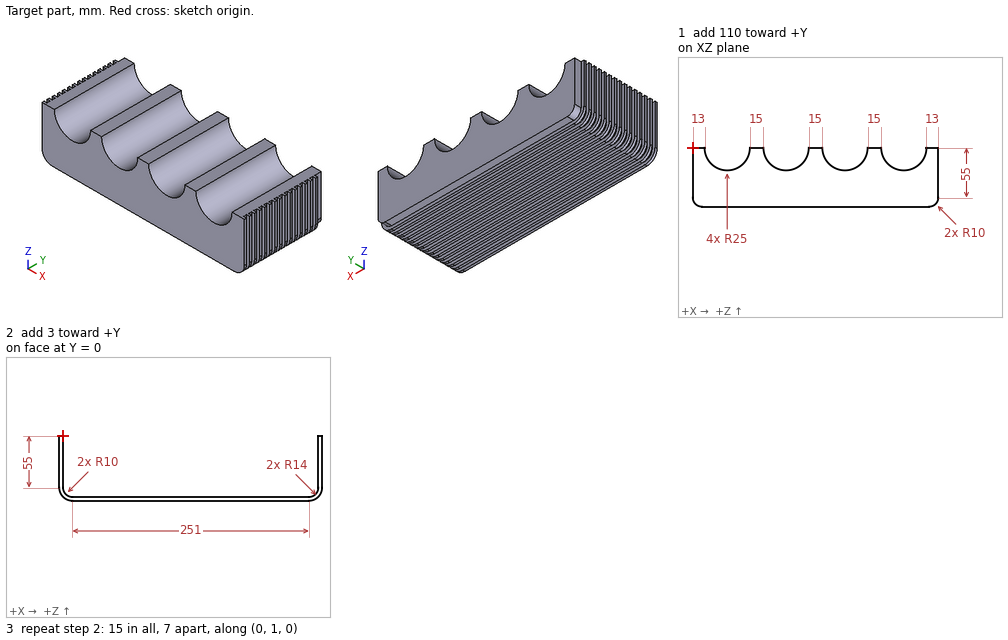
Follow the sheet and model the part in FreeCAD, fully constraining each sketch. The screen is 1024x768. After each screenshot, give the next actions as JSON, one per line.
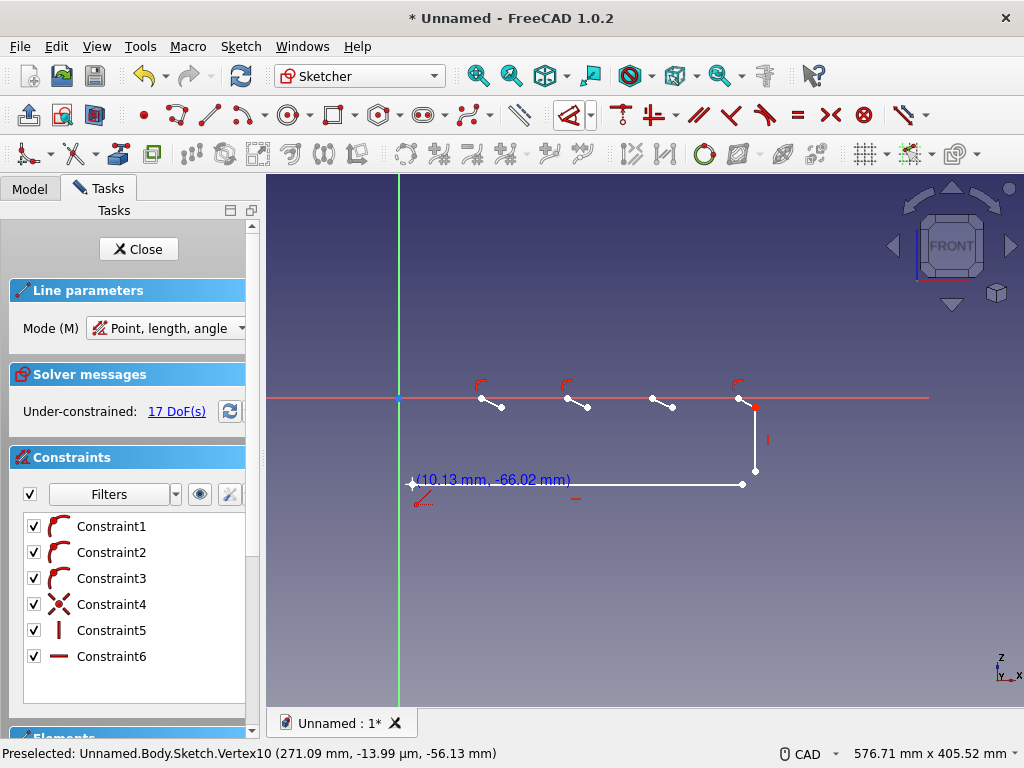
{"action": "key", "text": "g m"}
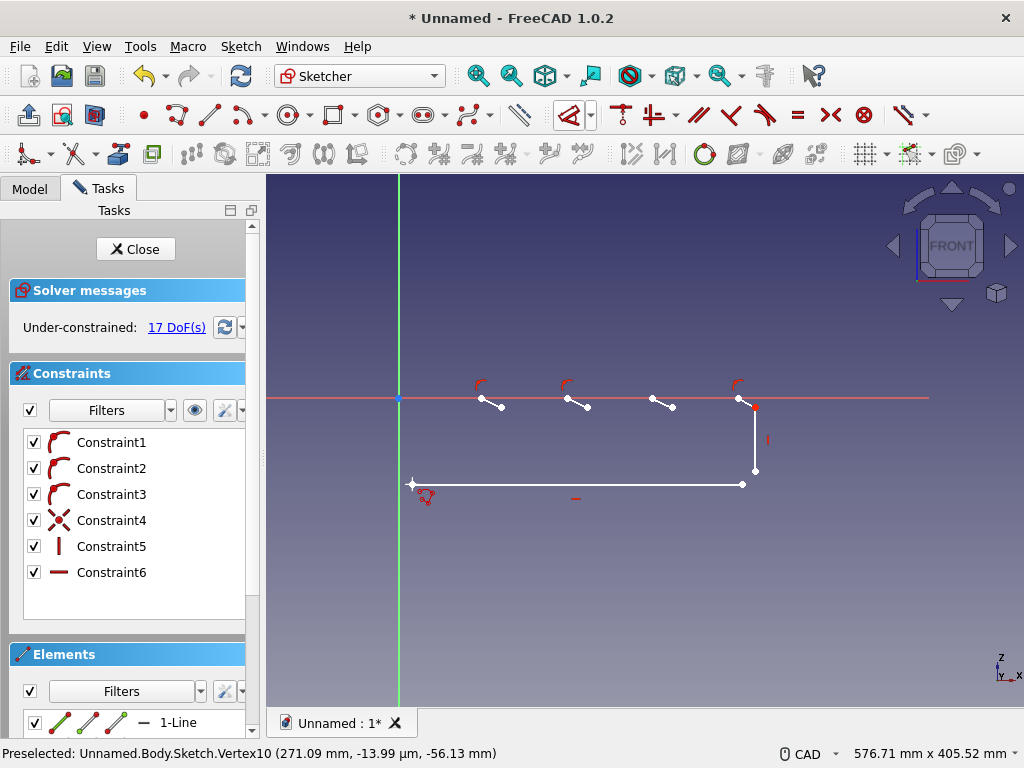
{"action": "left_click", "coordinate": [399, 471]}
{"action": "left_click", "coordinate": [399, 398]}
{"action": "left_click", "coordinate": [416, 407]}
{"action": "right_click", "coordinate": [416, 407]}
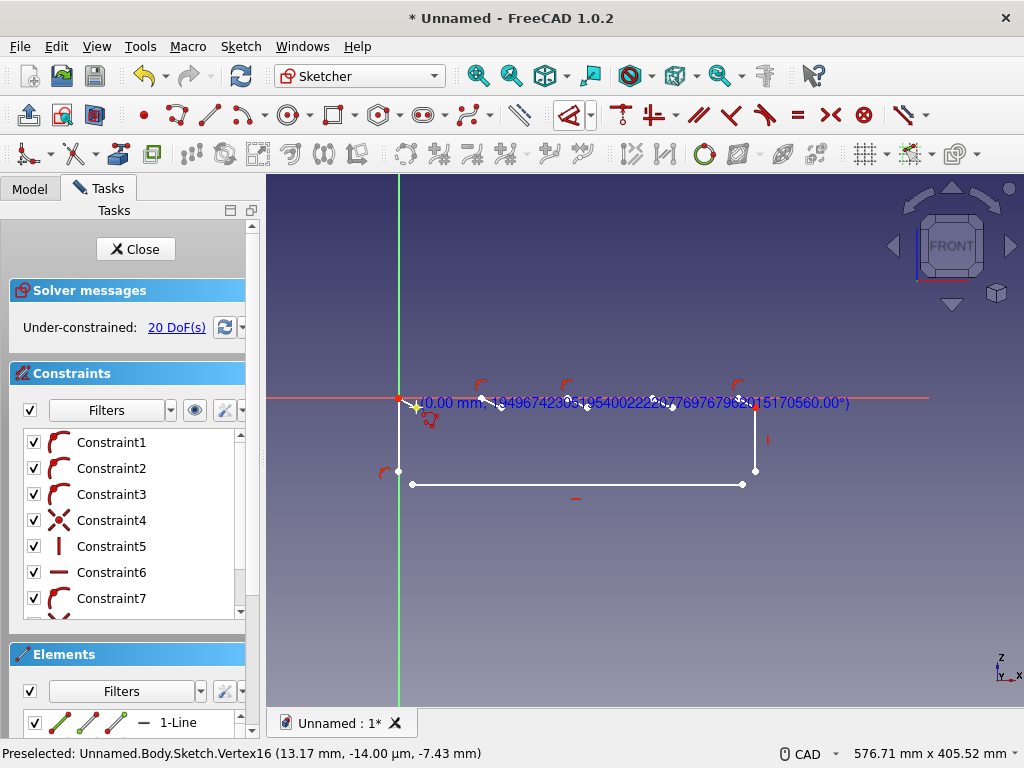
{"action": "key", "text": "g 3 a"}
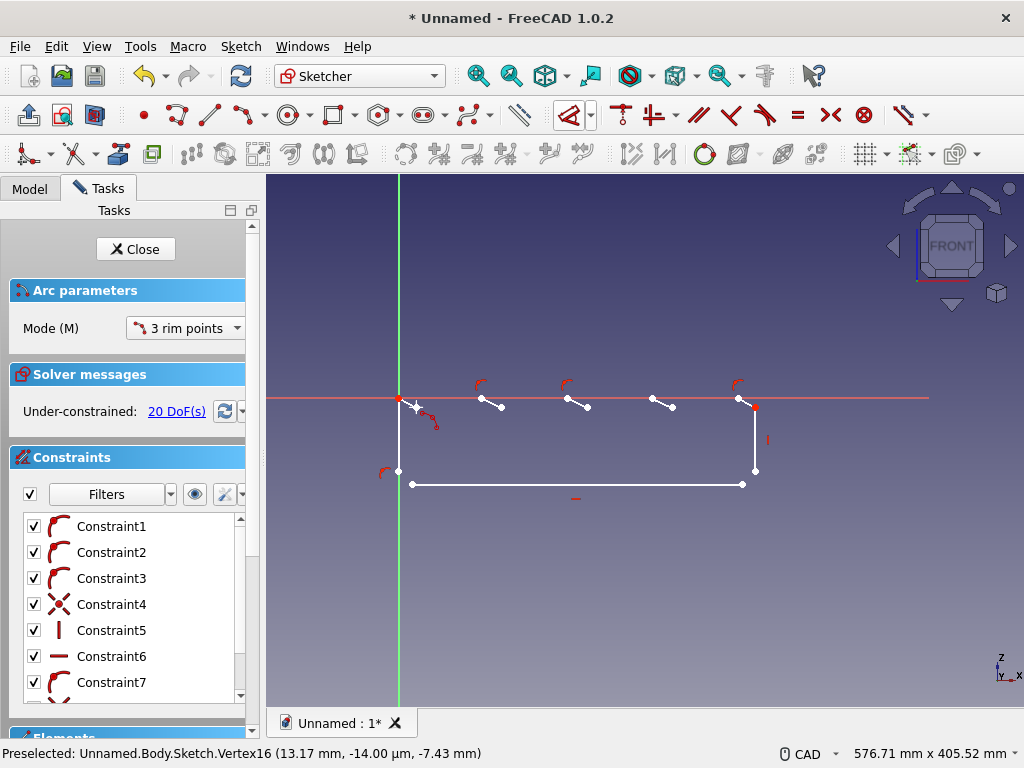
{"action": "scroll", "coordinate": [501, 398], "scroll_direction": "up", "scroll_amount": 3}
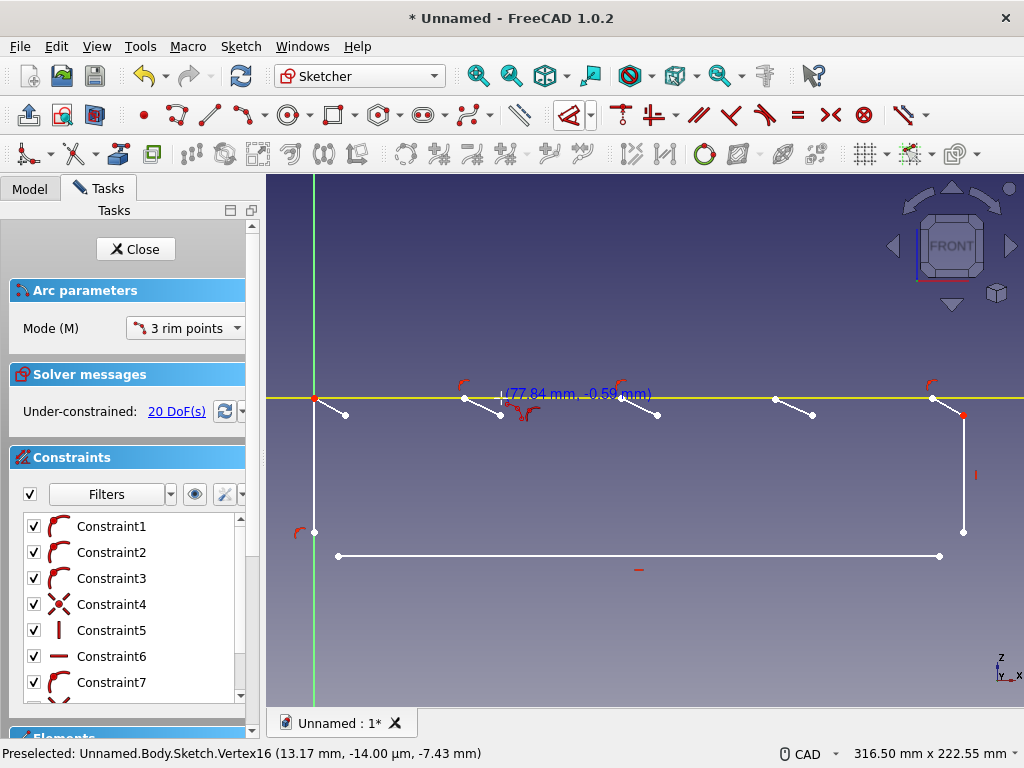
{"action": "left_click", "coordinate": [501, 416]}
{"action": "left_click", "coordinate": [621, 398]}
{"action": "left_click", "coordinate": [561, 458]}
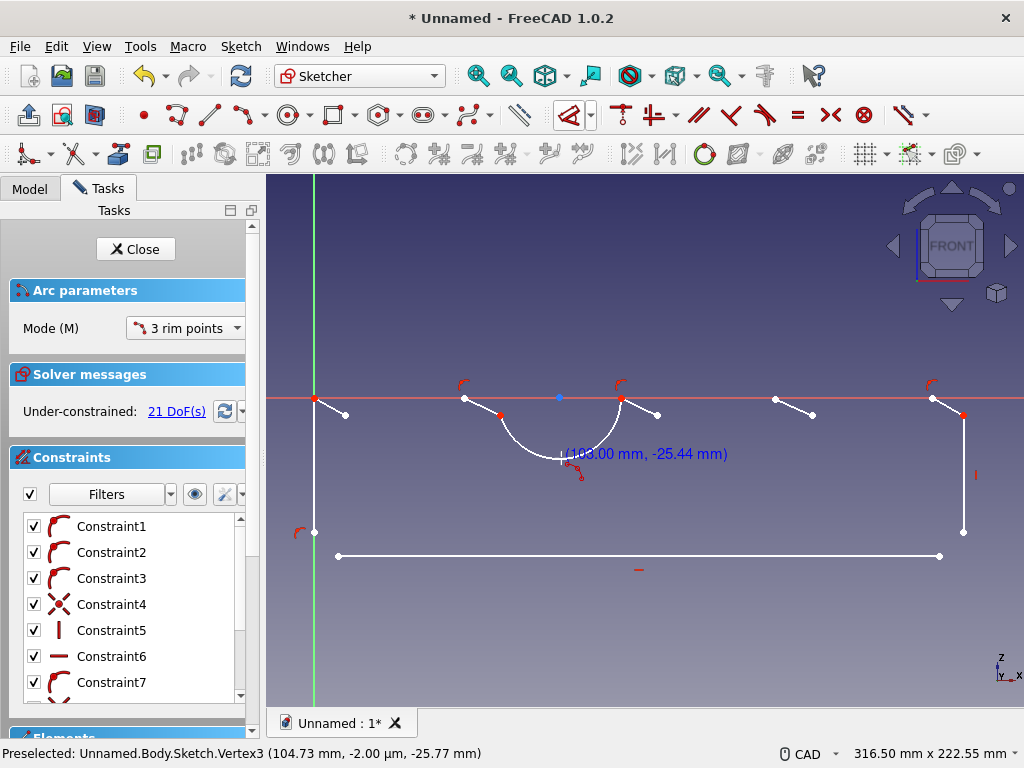
{"action": "left_click", "coordinate": [657, 416]}
{"action": "left_click", "coordinate": [776, 399]}
{"action": "left_click", "coordinate": [717, 458]}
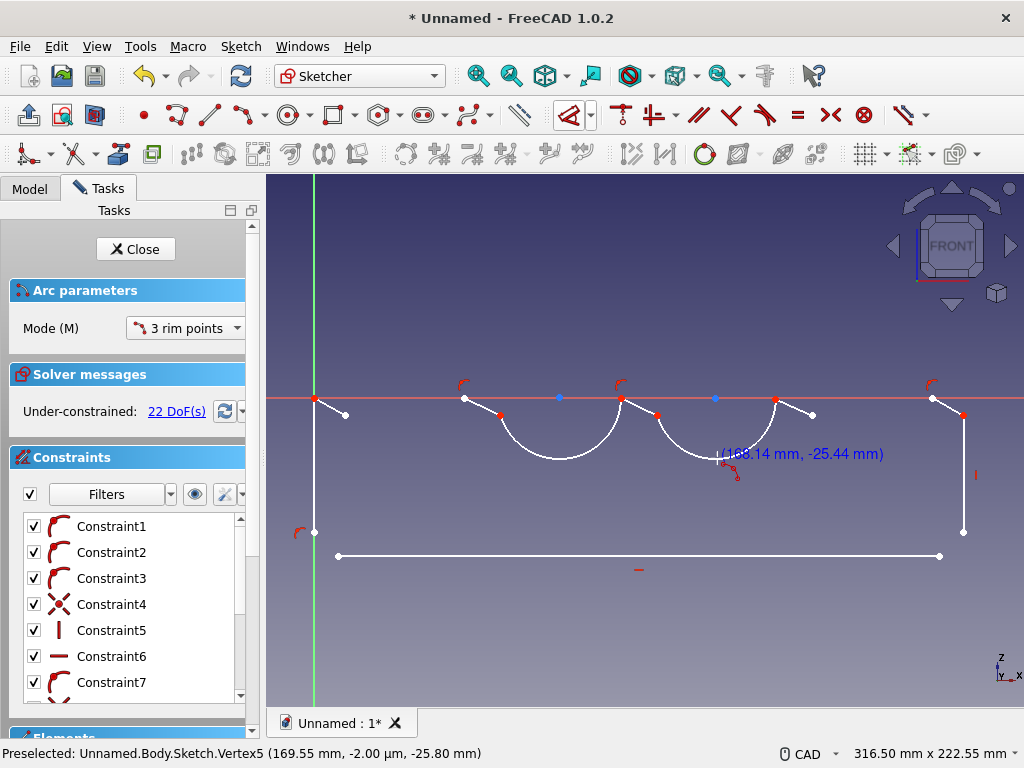
{"action": "left_click", "coordinate": [812, 416]}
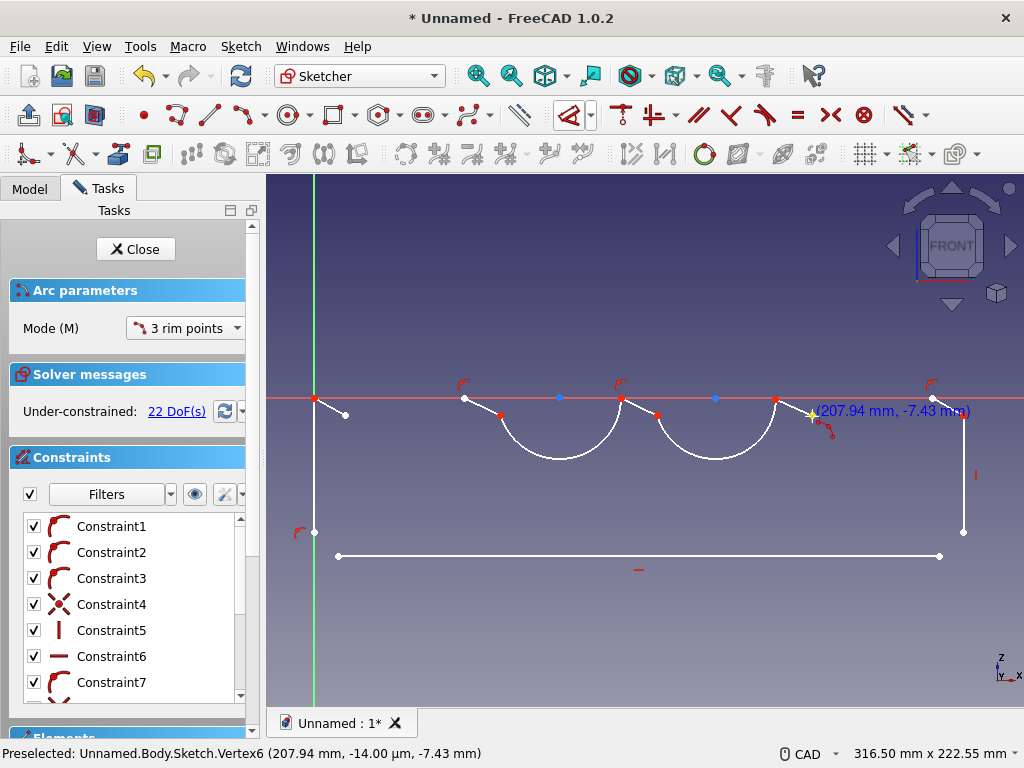
{"action": "scroll", "coordinate": [450, 369], "scroll_direction": "down", "scroll_amount": 2}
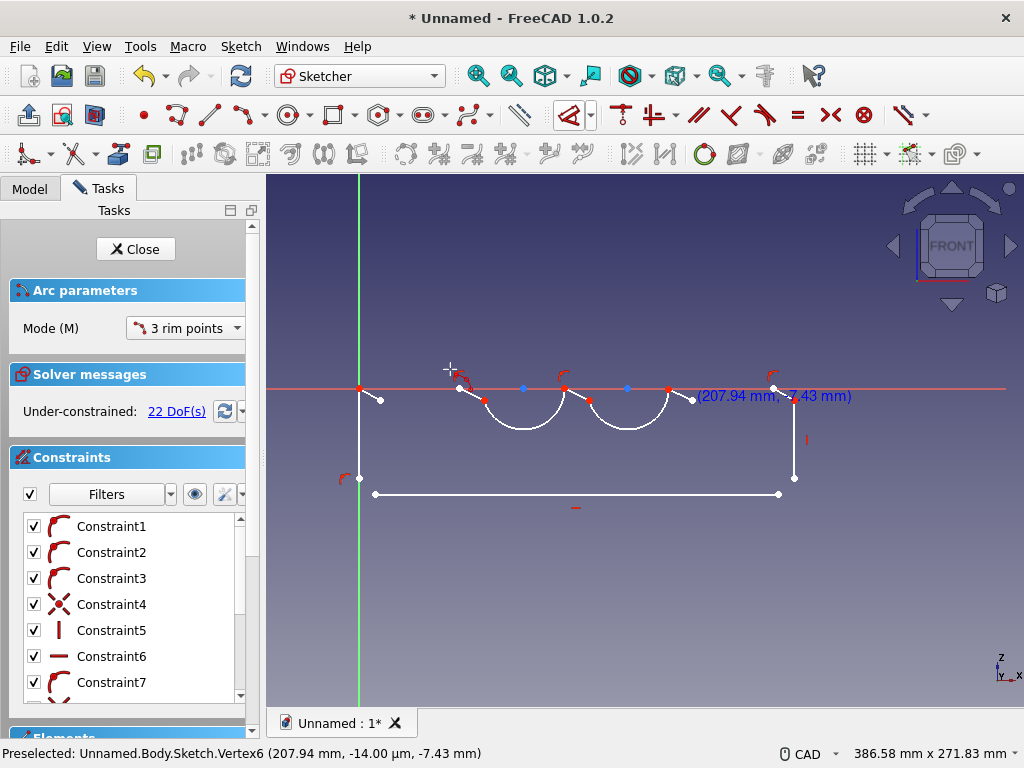
{"action": "scroll", "coordinate": [773, 389], "scroll_direction": "up", "scroll_amount": 3}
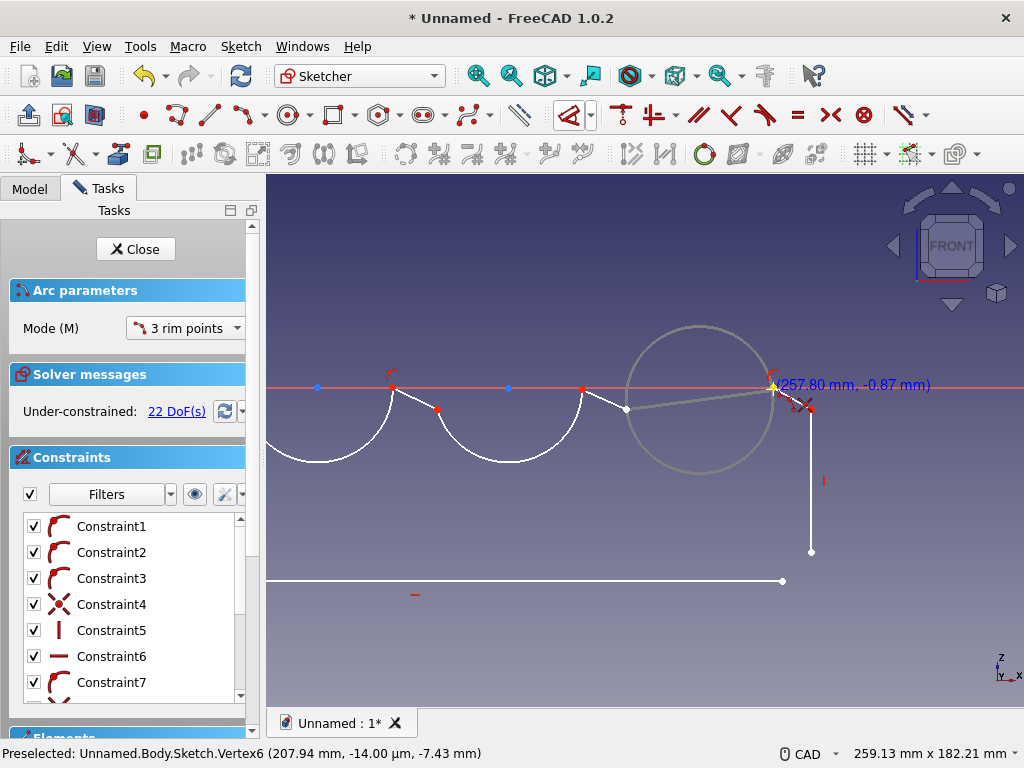
{"action": "left_click", "coordinate": [773, 388]}
{"action": "left_click", "coordinate": [700, 461]}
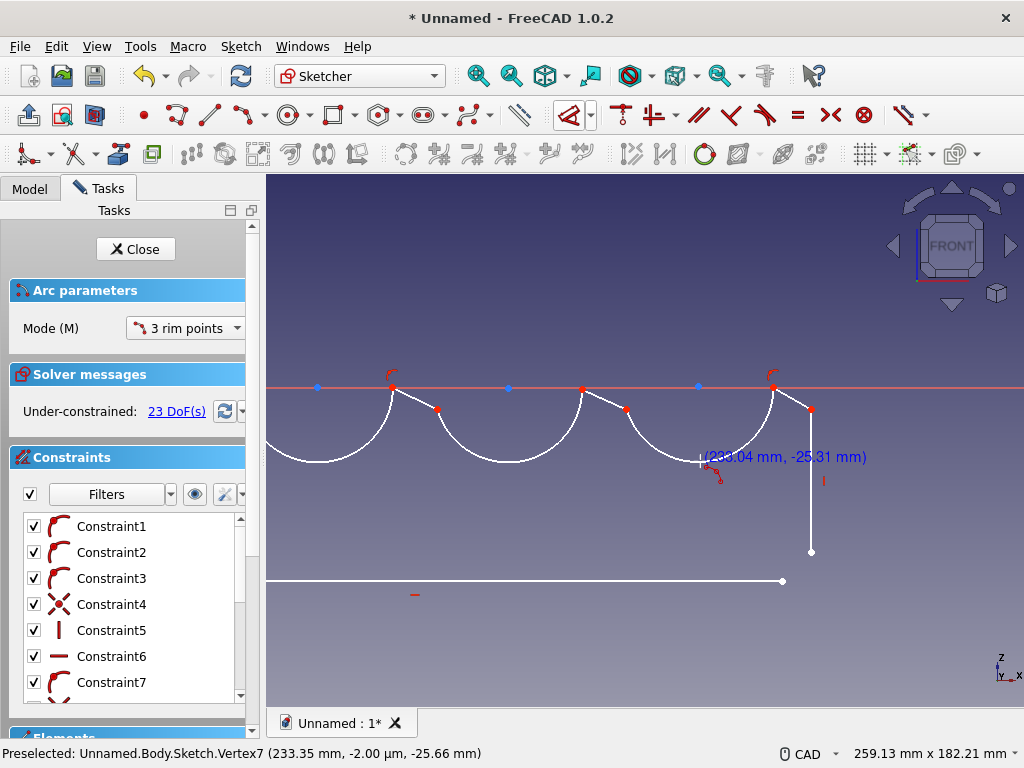
{"action": "left_click", "coordinate": [811, 552]}
{"action": "left_click", "coordinate": [782, 581]}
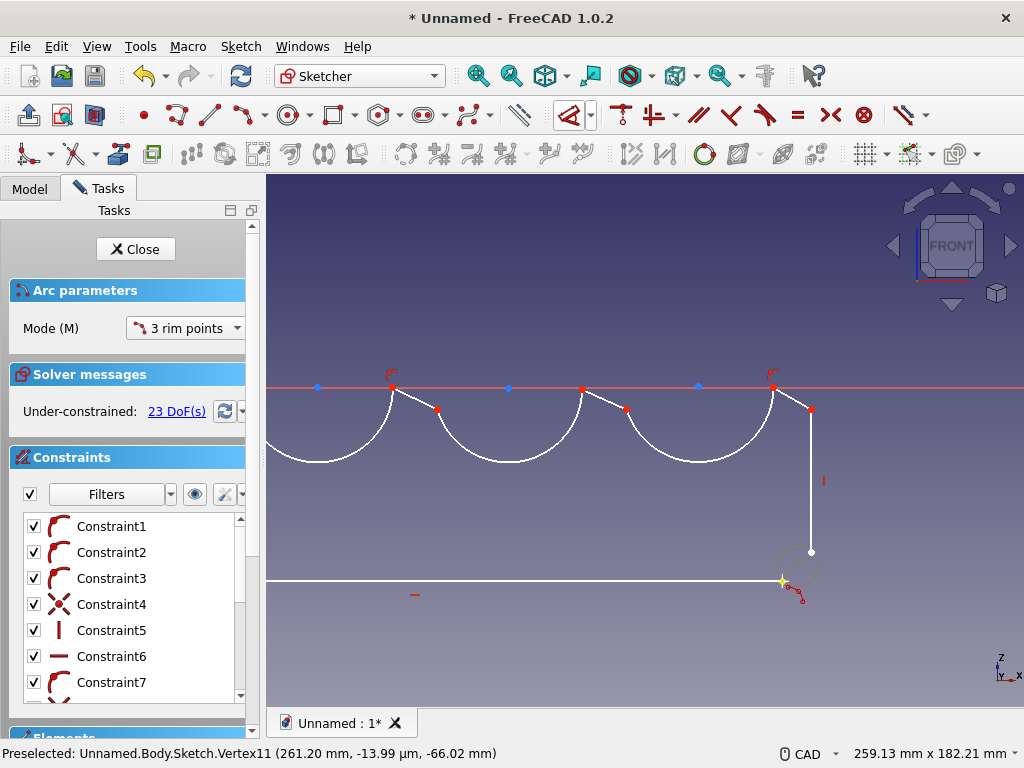
{"action": "scroll", "coordinate": [802, 570], "scroll_direction": "up", "scroll_amount": 4}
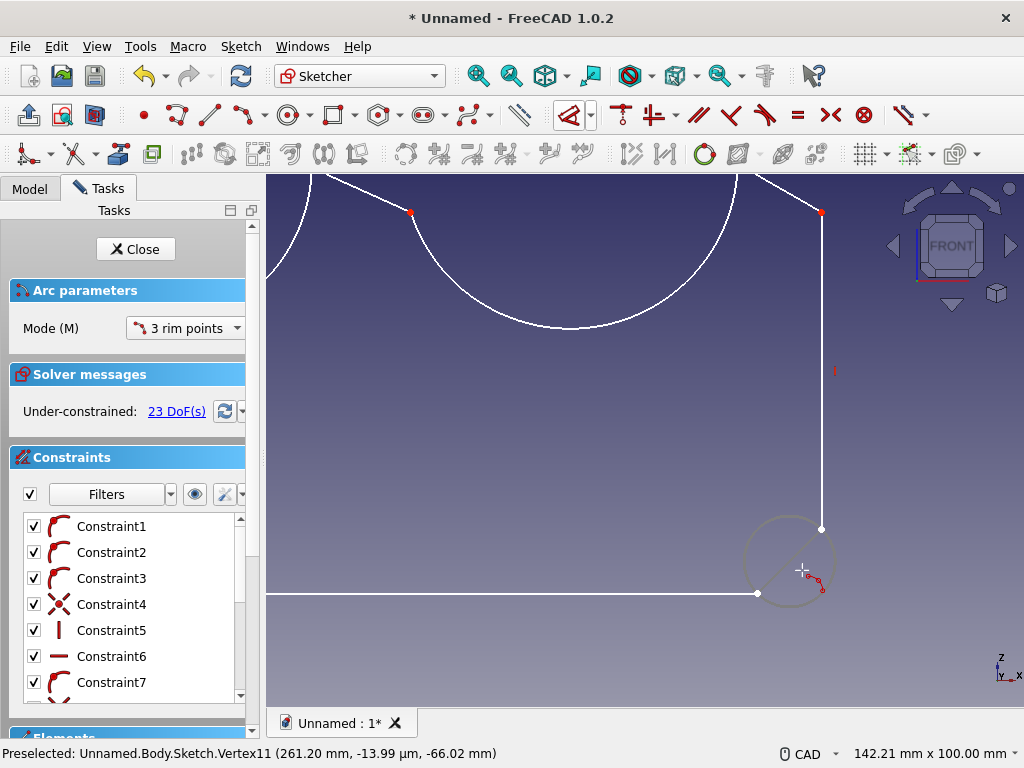
{"action": "left_click", "coordinate": [802, 568]}